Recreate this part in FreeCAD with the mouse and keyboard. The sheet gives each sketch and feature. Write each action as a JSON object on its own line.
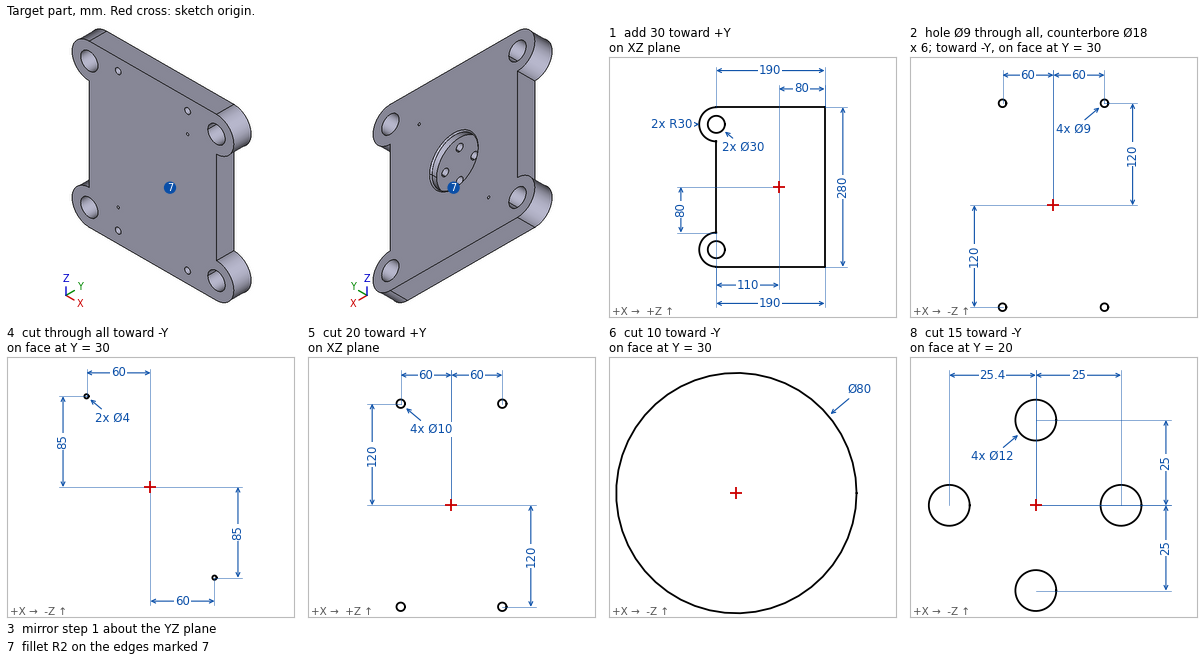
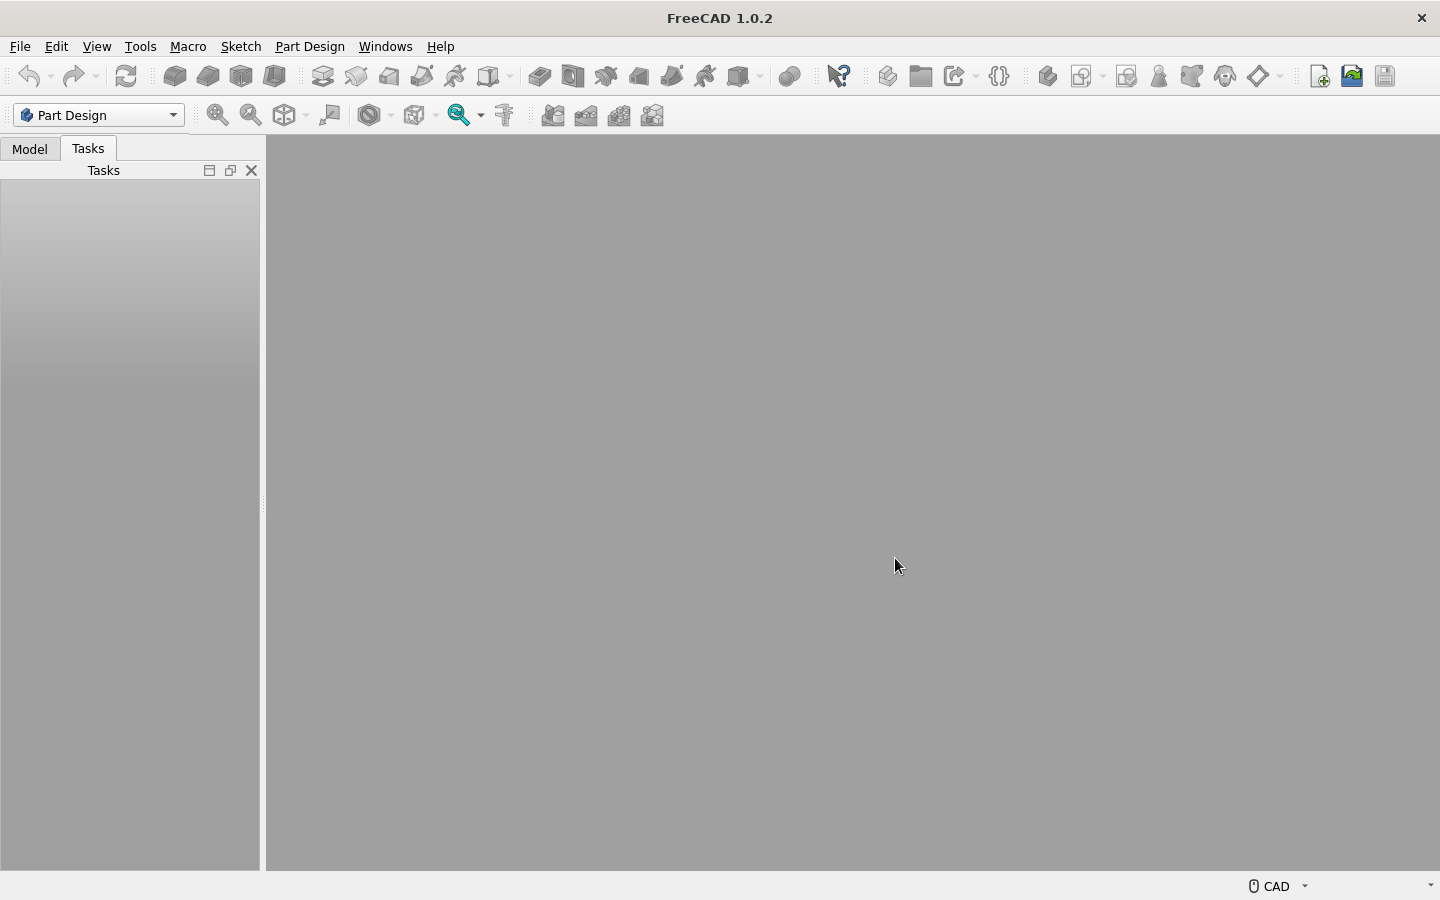
{"action": "left_click", "coordinate": [1319, 76]}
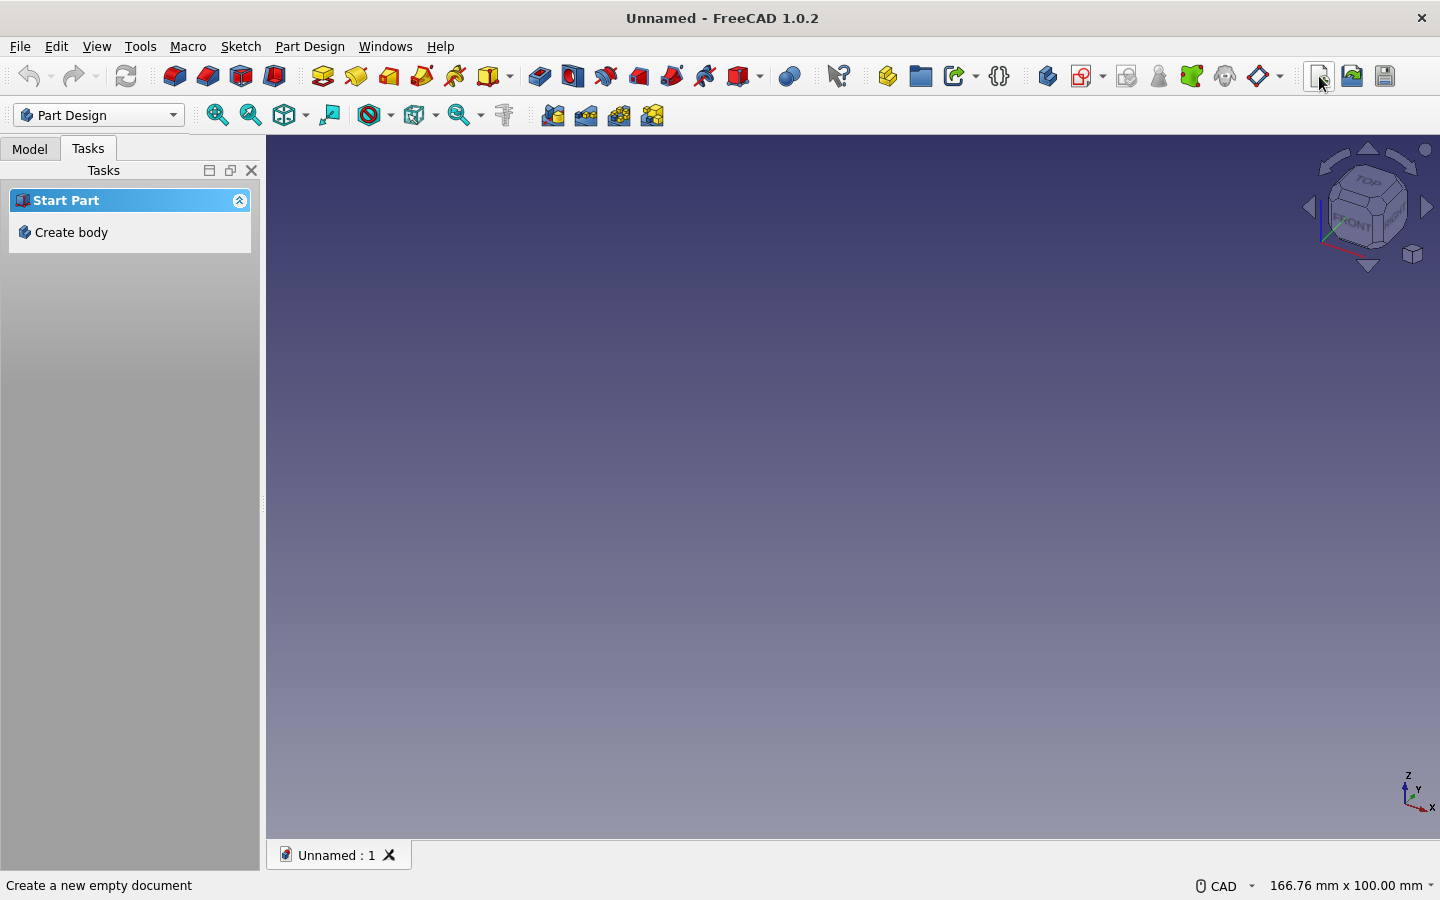
{"action": "left_click", "coordinate": [1080, 76]}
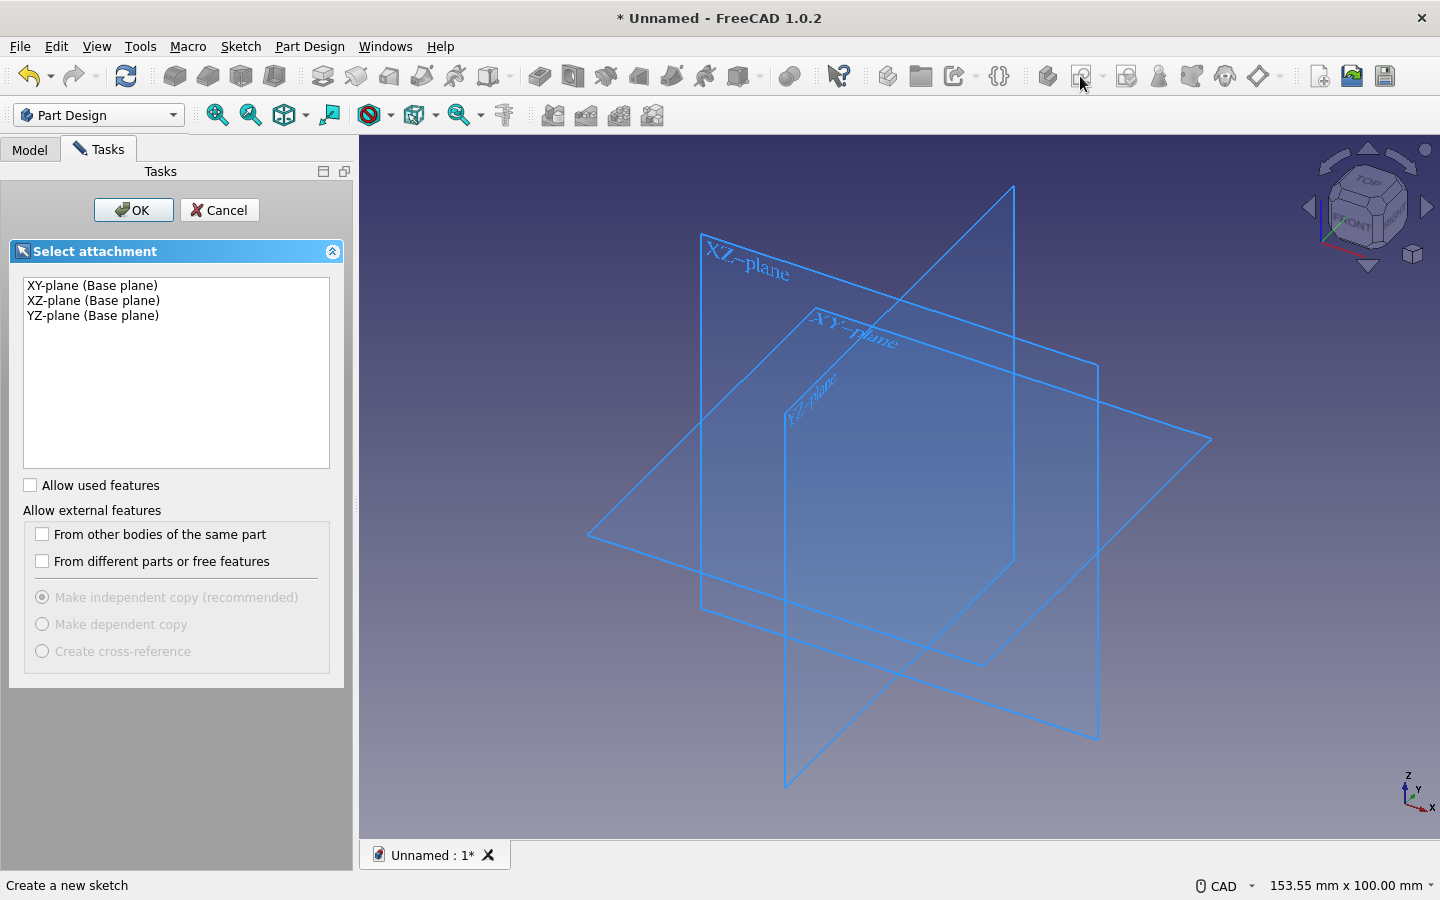
{"action": "left_click", "coordinate": [84, 300]}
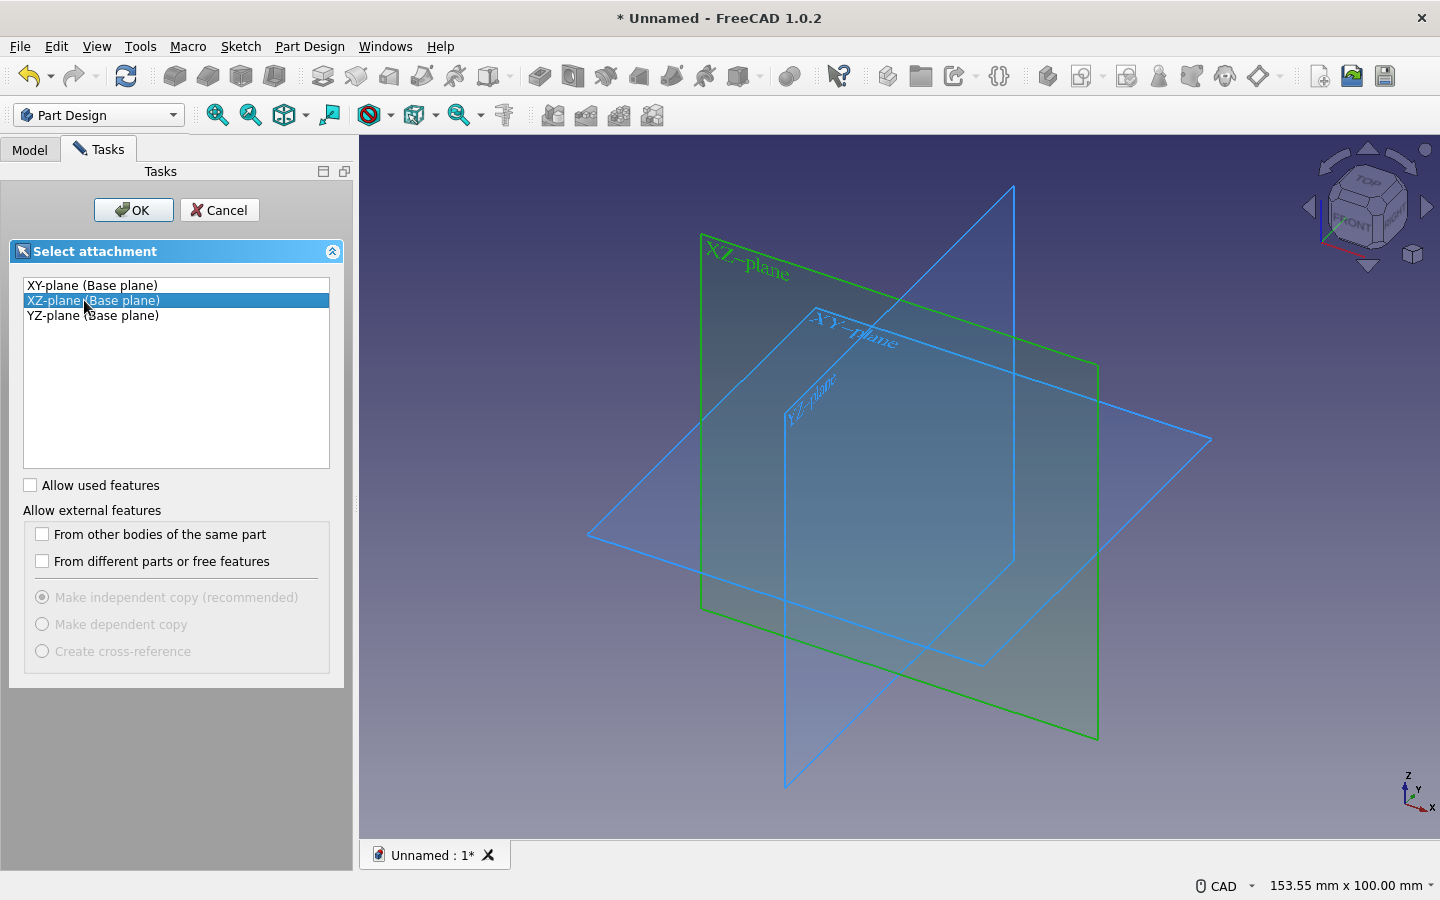
{"action": "left_click", "coordinate": [134, 210]}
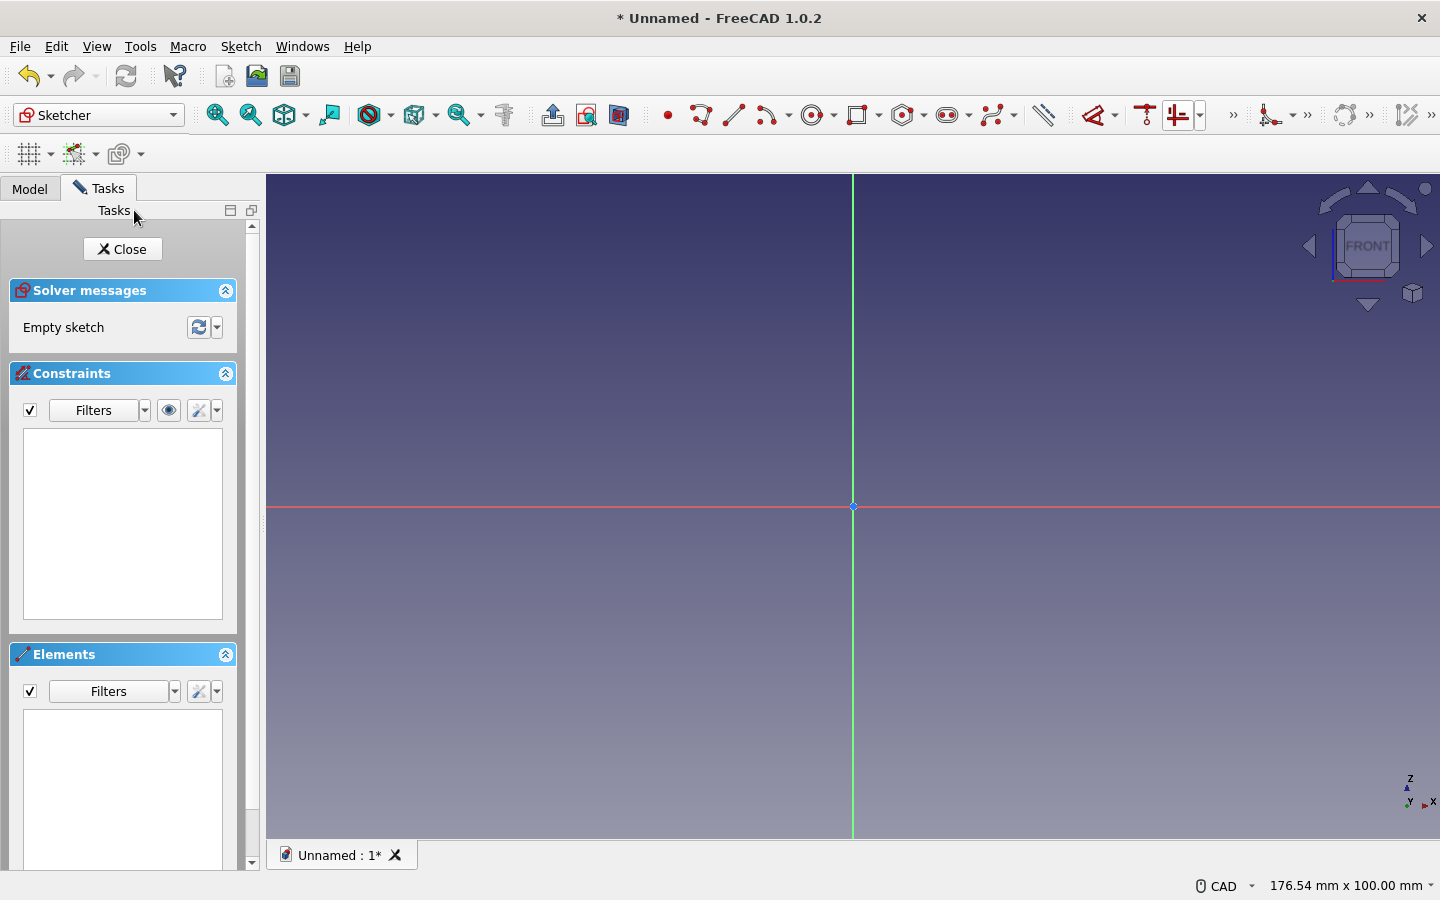
{"action": "scroll", "coordinate": [827, 506], "scroll_direction": "down", "scroll_amount": 7}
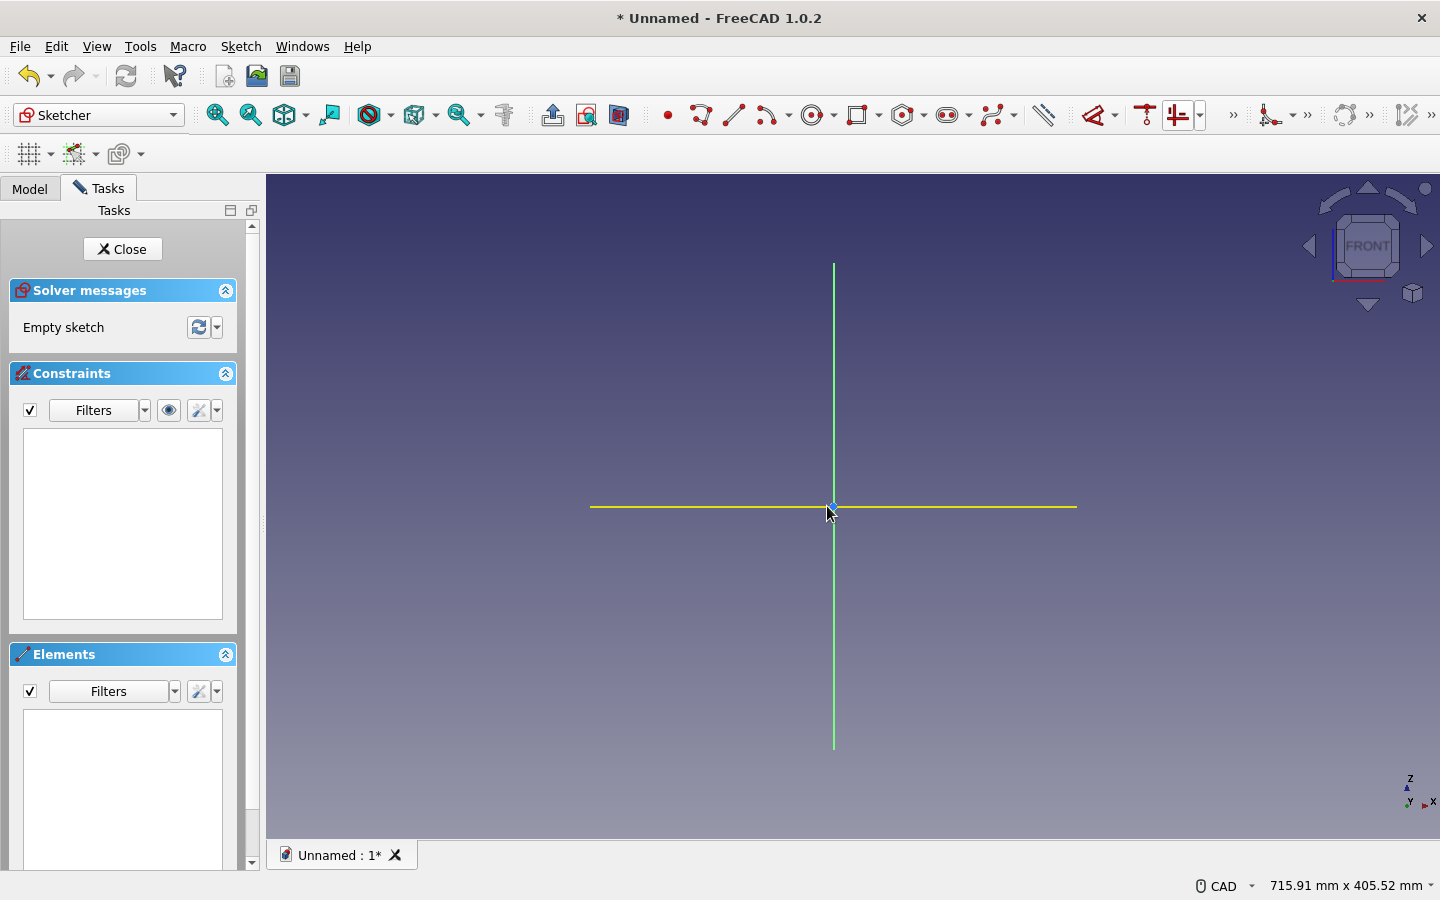
{"action": "left_click", "coordinate": [701, 116]}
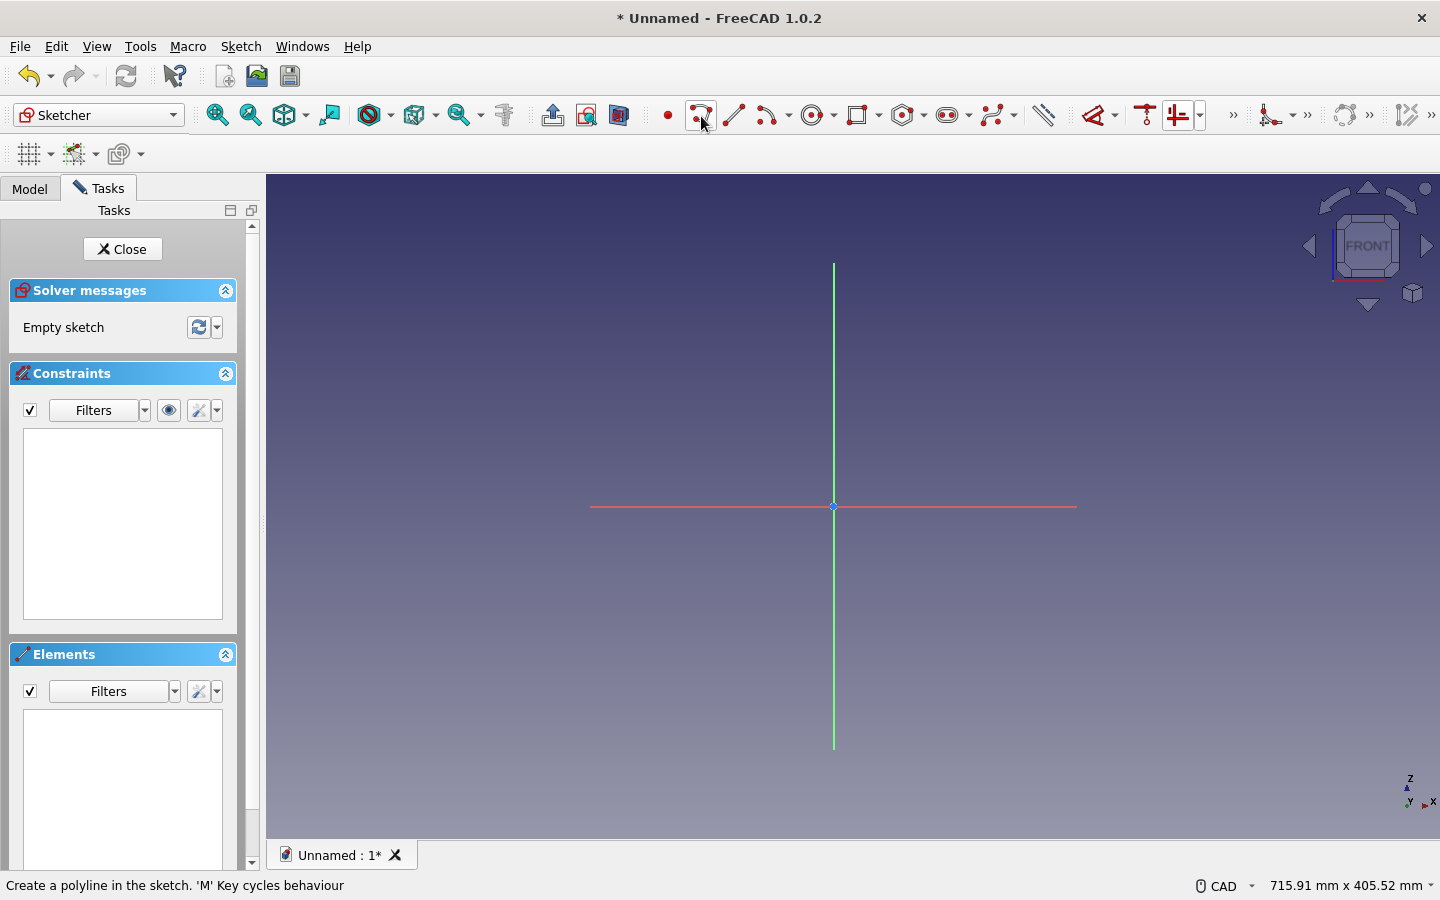
{"action": "left_click", "coordinate": [653, 277]}
{"action": "left_click", "coordinate": [965, 277]}
{"action": "left_click", "coordinate": [965, 736]}
{"action": "left_click", "coordinate": [653, 736]}
{"action": "right_click", "coordinate": [653, 736]}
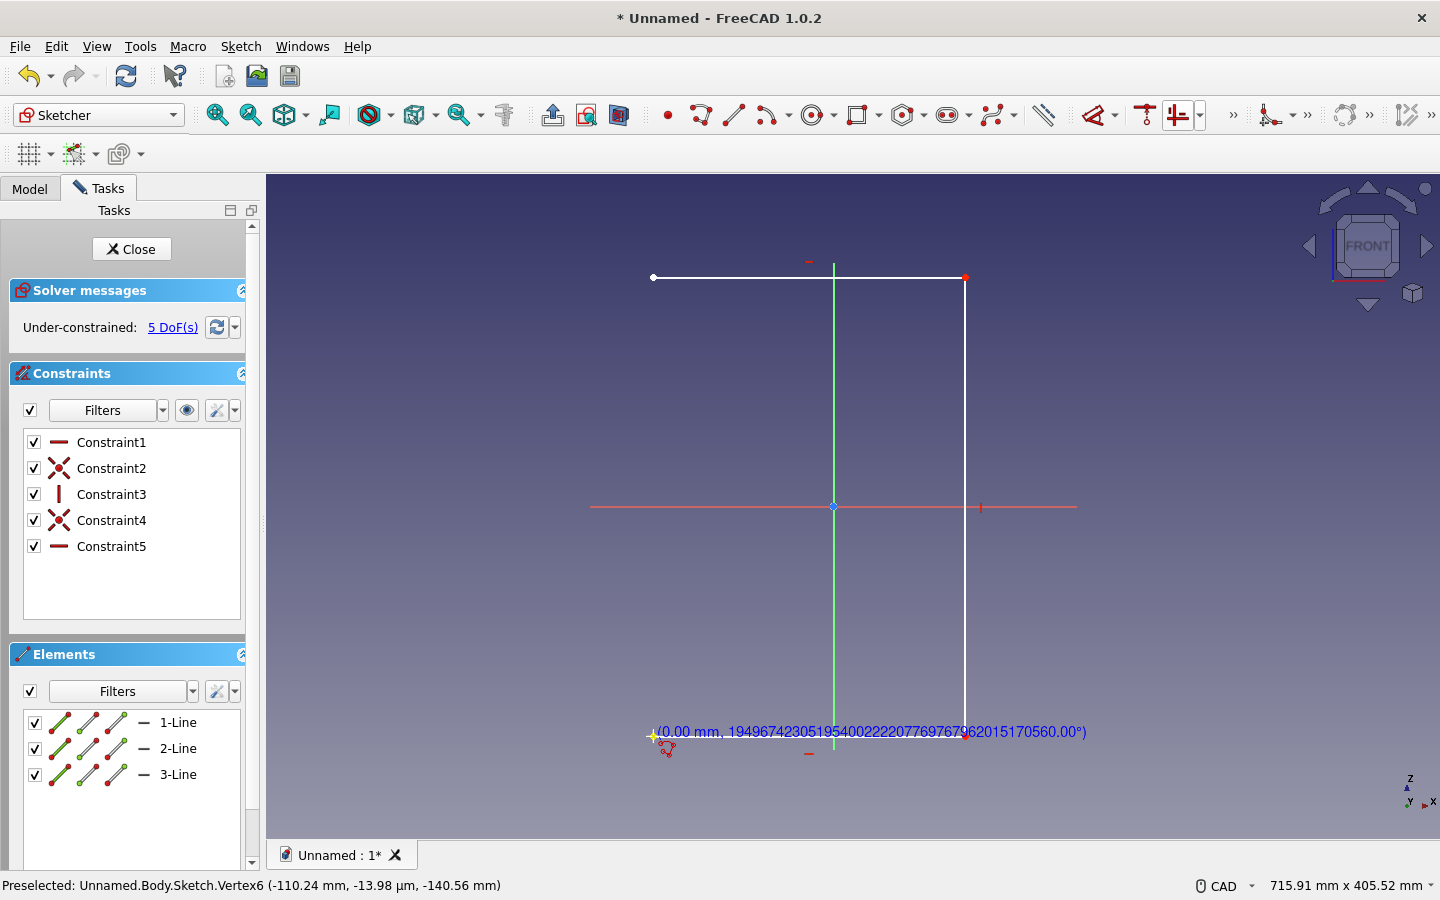
{"action": "key", "text": "g l"}